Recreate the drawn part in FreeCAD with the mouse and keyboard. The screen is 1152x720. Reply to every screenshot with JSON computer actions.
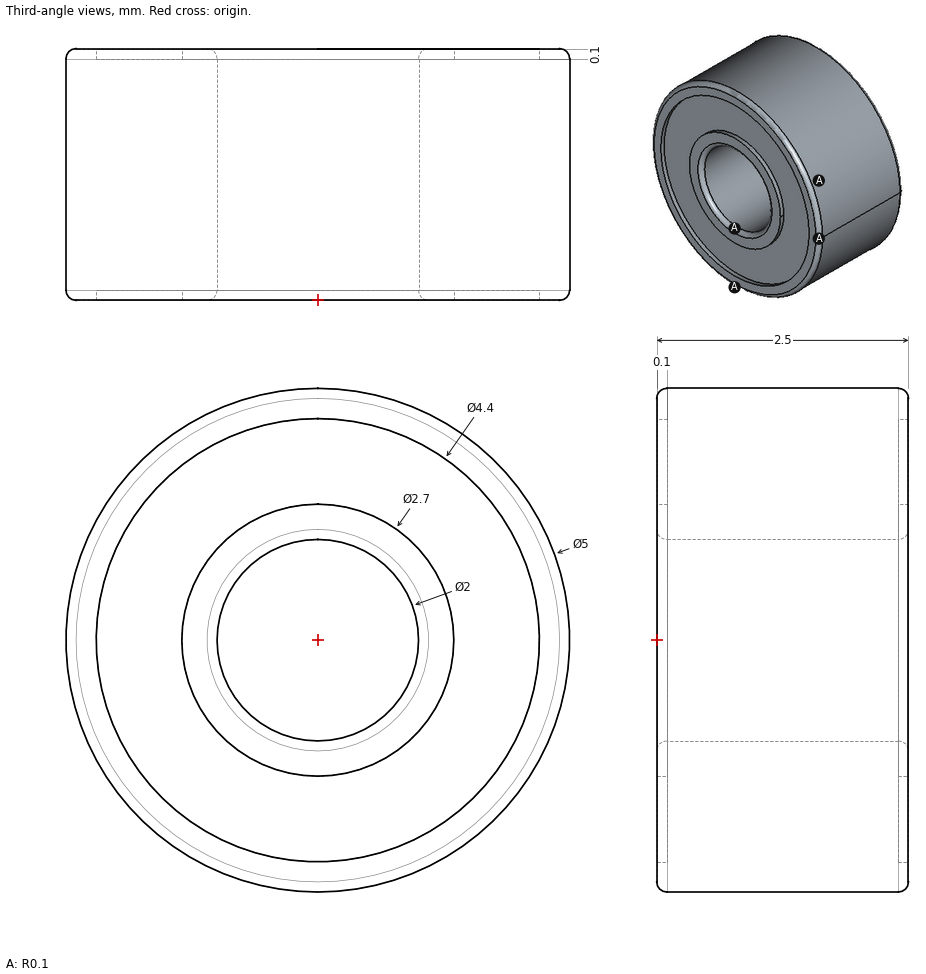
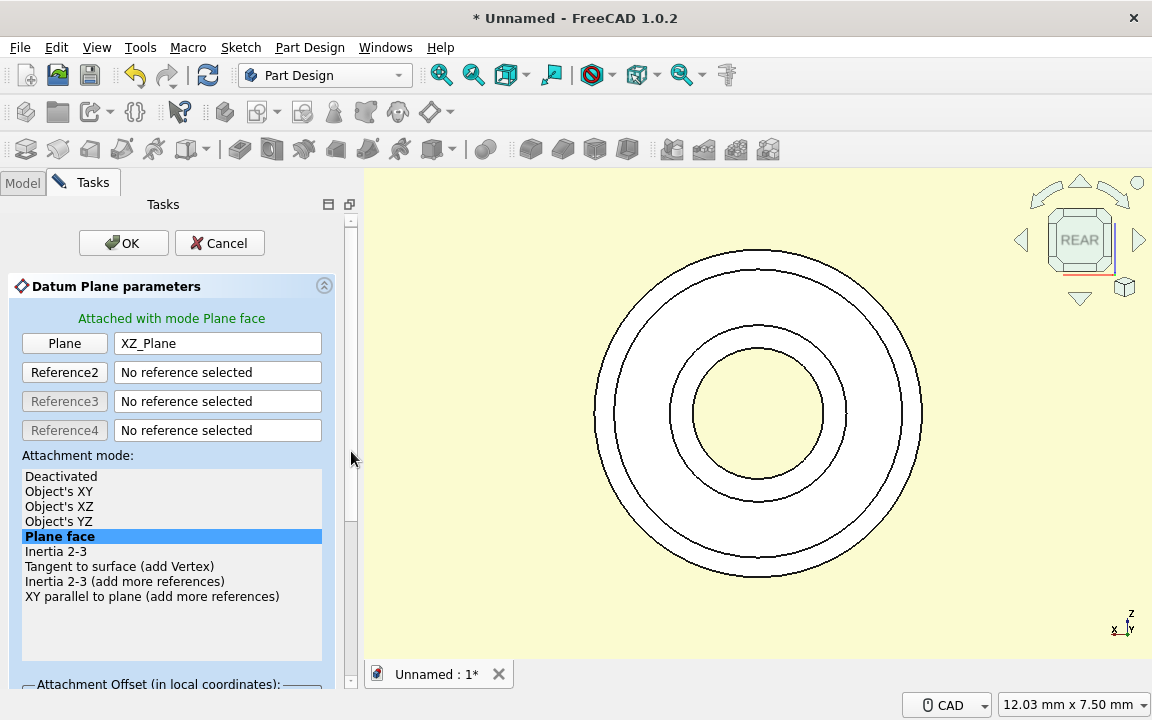
{"action": "left_click", "coordinate": [124, 243]}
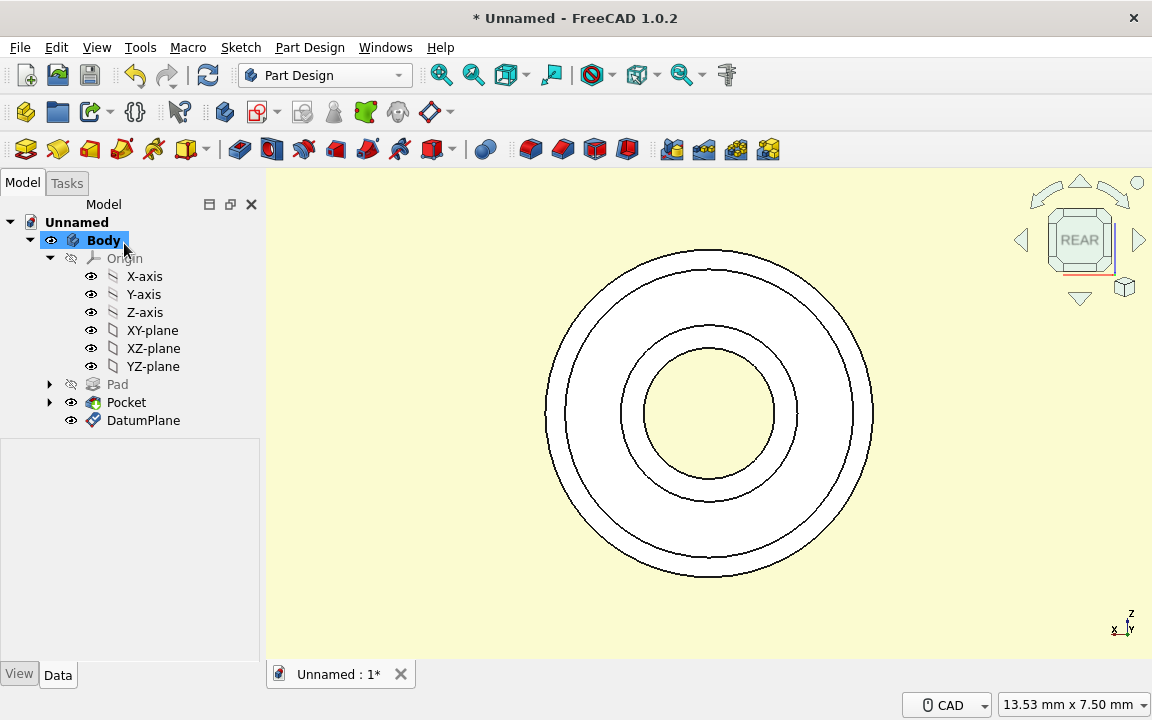
{"action": "left_click", "coordinate": [116, 420]}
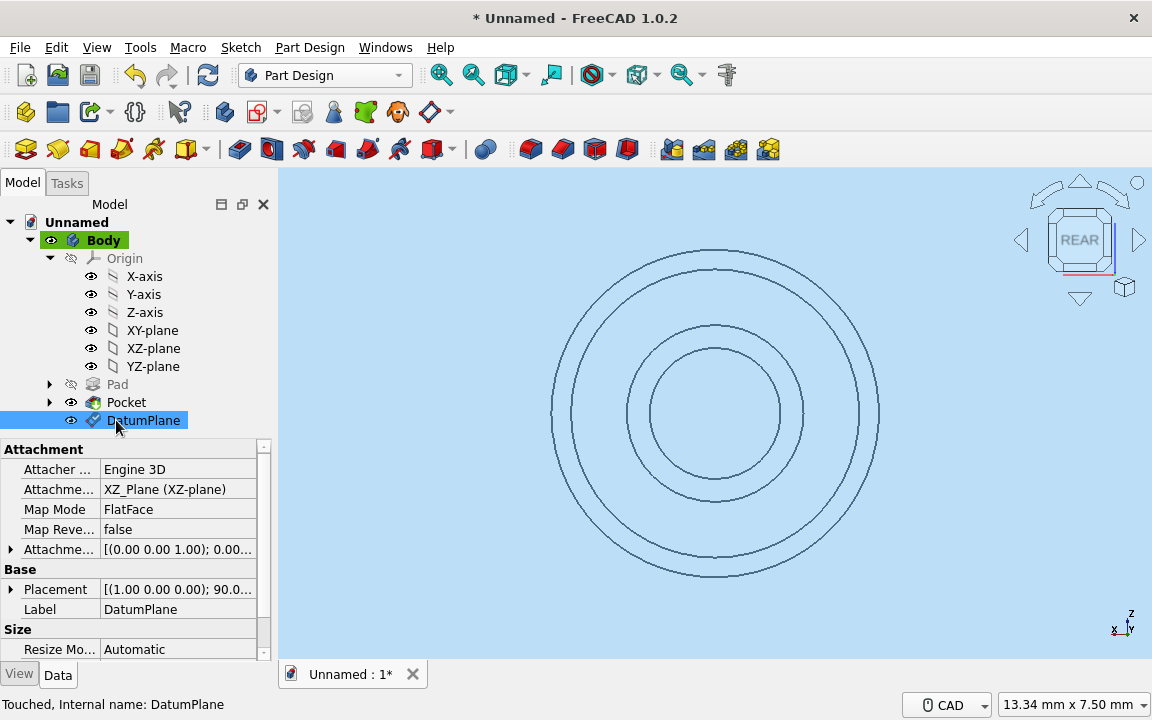
{"action": "left_click", "coordinate": [258, 112]}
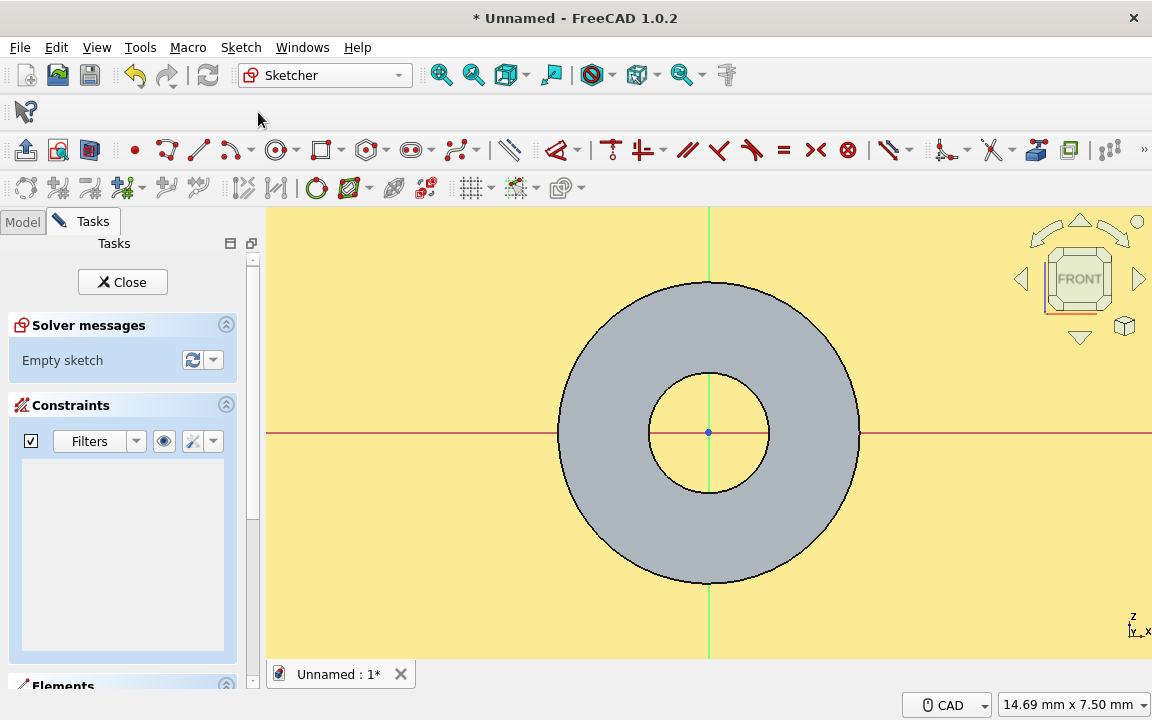
{"action": "left_click", "coordinate": [90, 150]}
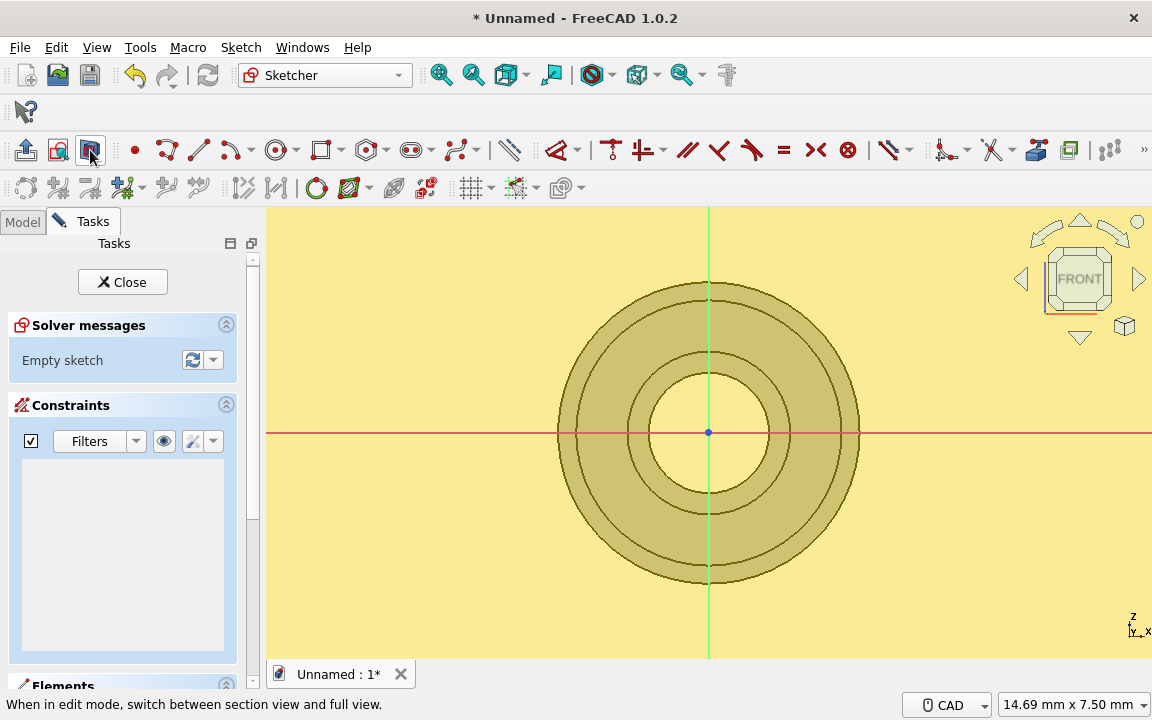
{"action": "key", "text": "g c"}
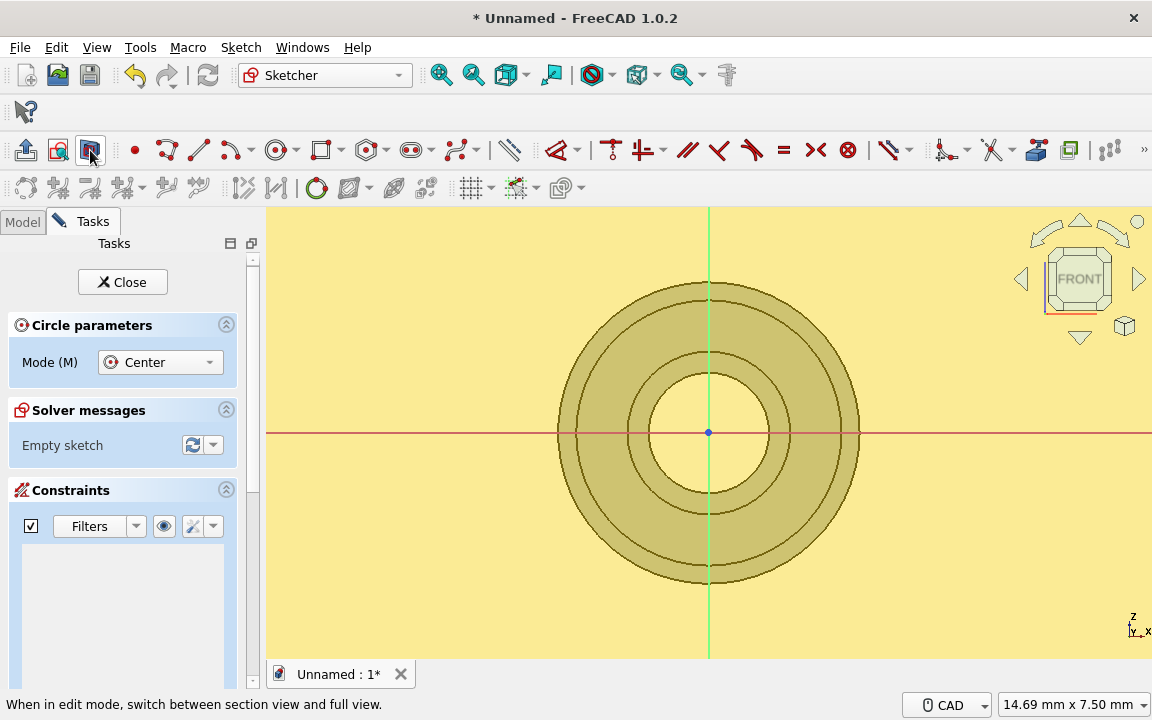
{"action": "left_click", "coordinate": [709, 433]}
{"action": "mouse_move", "coordinate": [803, 339]}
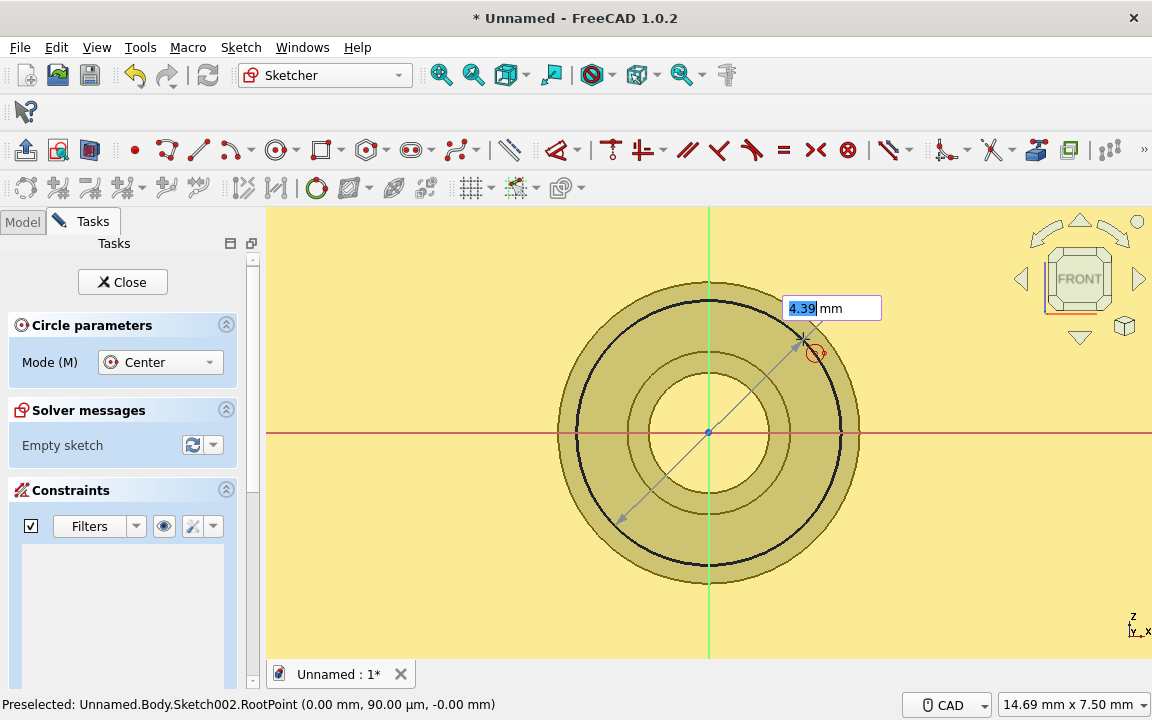
{"action": "type", "text": "4.4"}
{"action": "key", "text": "Return"}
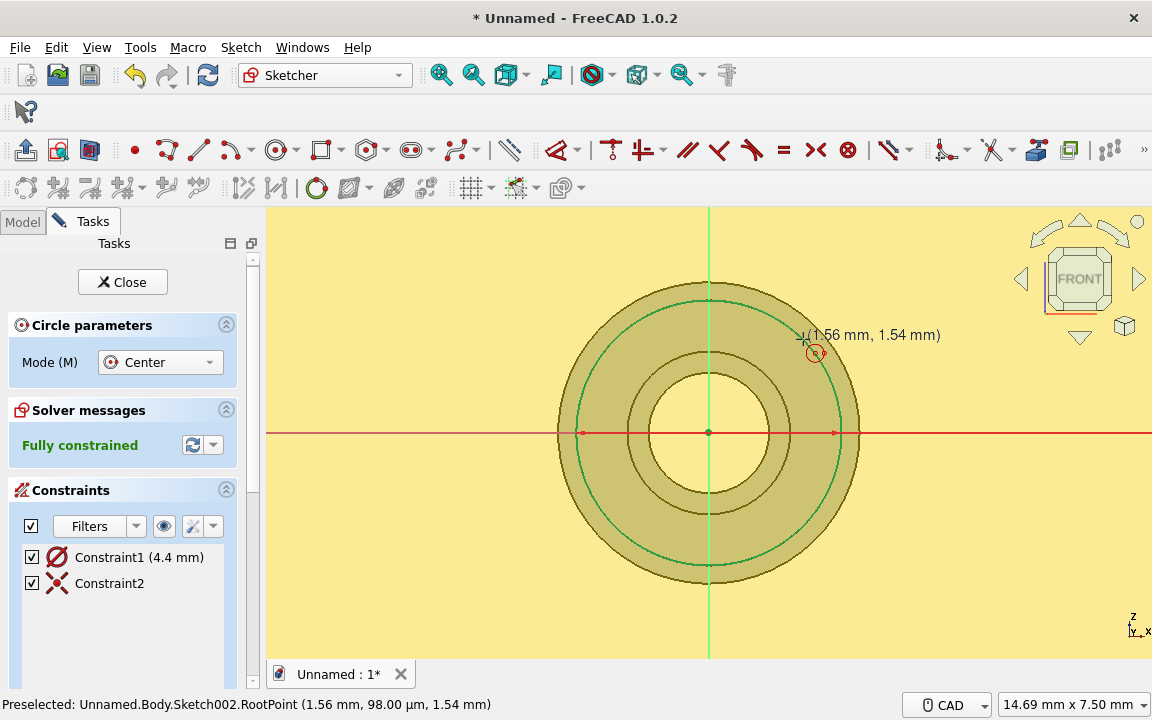
{"action": "left_click", "coordinate": [709, 433]}
{"action": "mouse_move", "coordinate": [766, 375]}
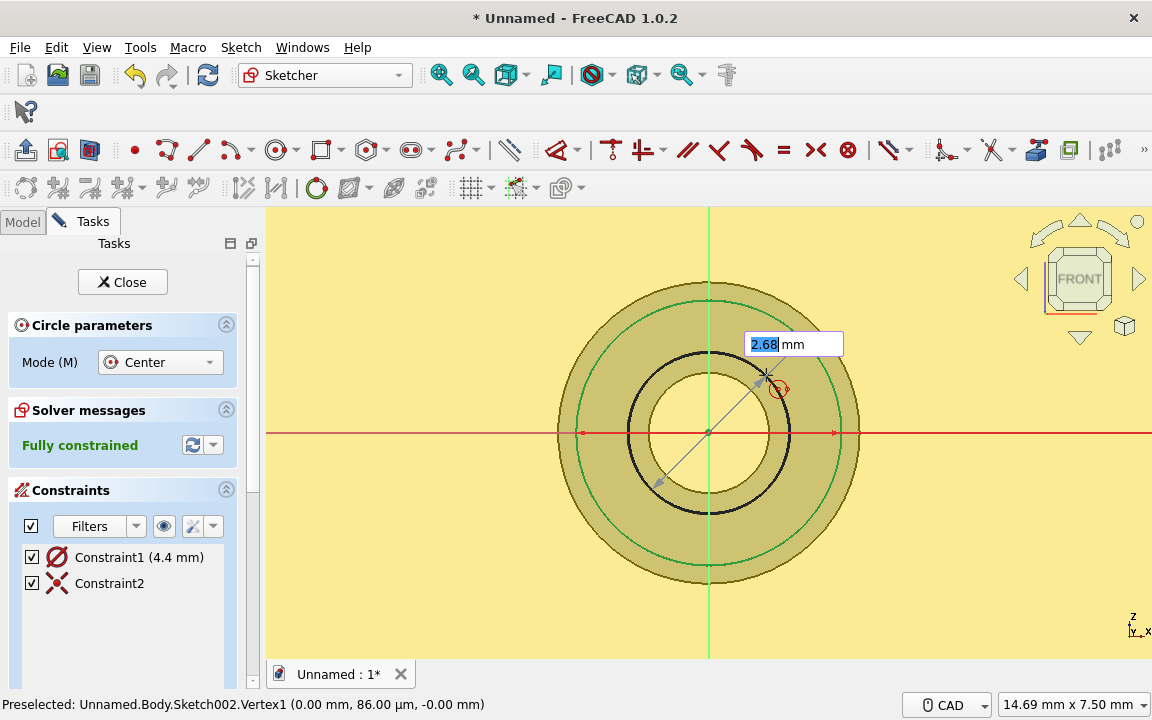
{"action": "type", "text": "2.7"}
{"action": "key", "text": "Return"}
{"action": "key", "text": "Escape"}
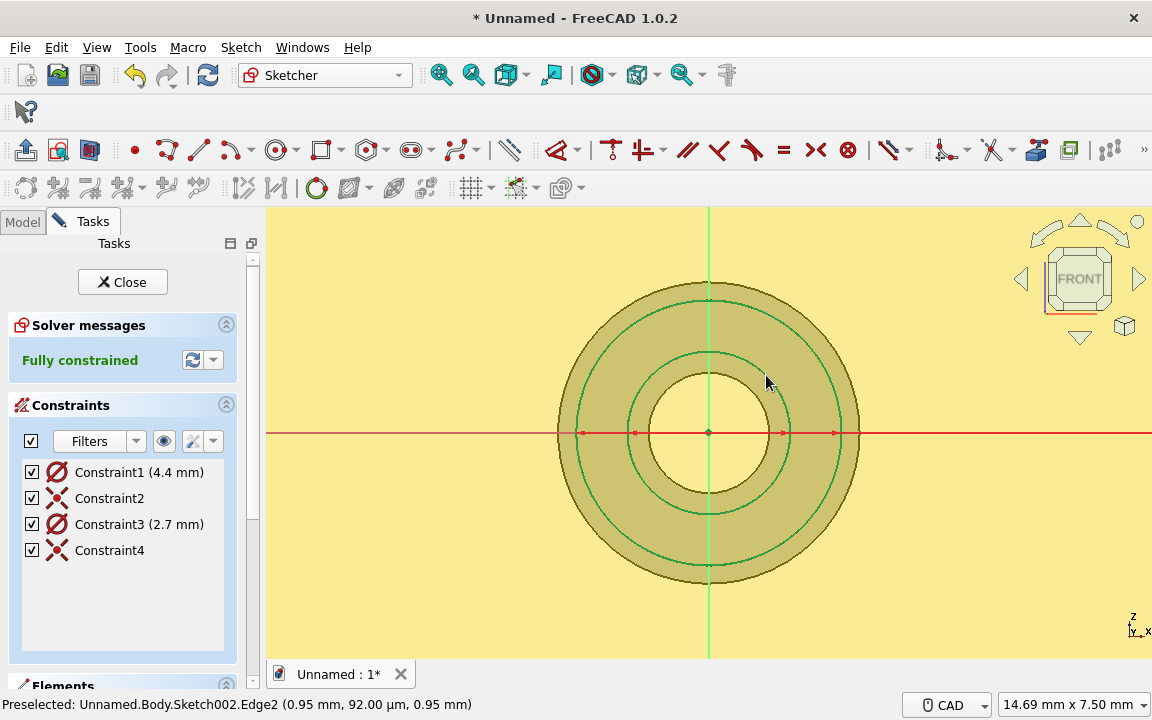
{"action": "left_click", "coordinate": [123, 282]}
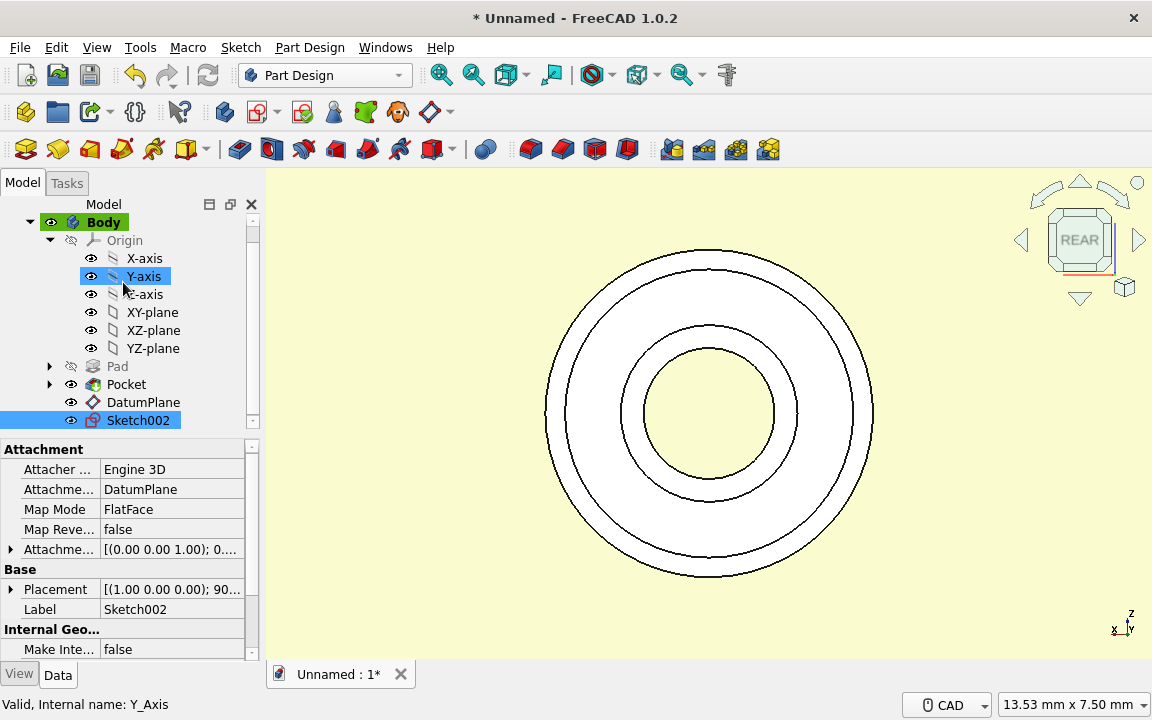
{"action": "left_click", "coordinate": [240, 150]}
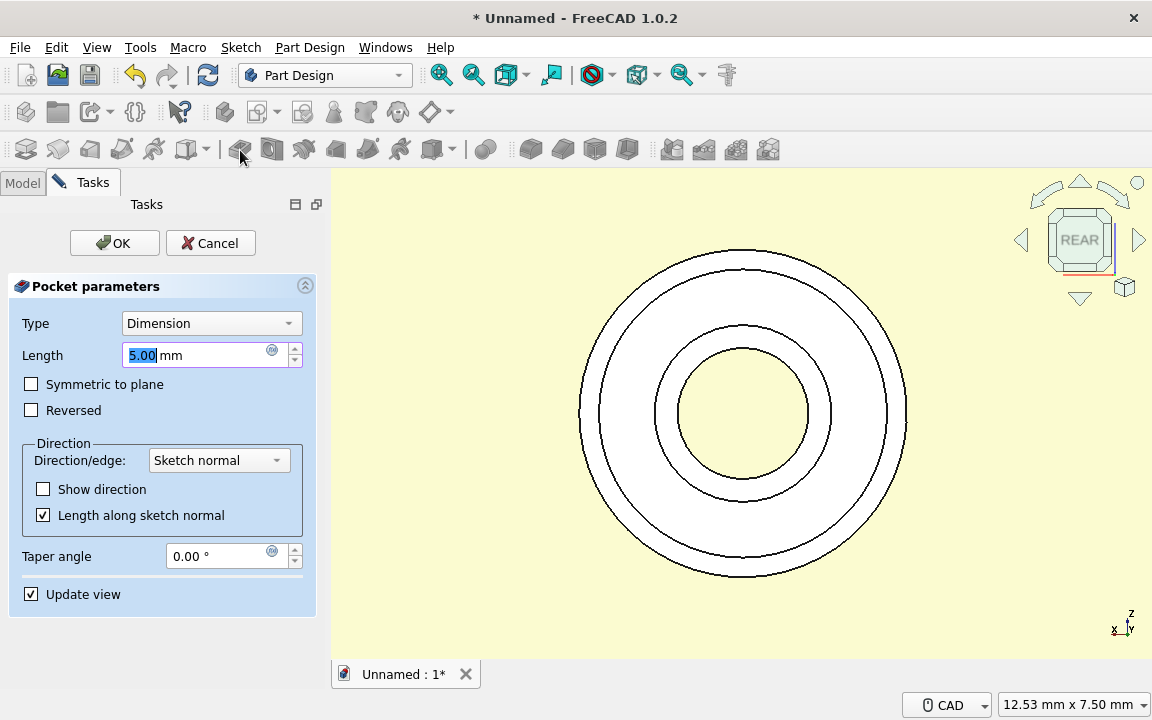
{"action": "type", "text": "0.1"}
{"action": "key", "text": "Tab"}